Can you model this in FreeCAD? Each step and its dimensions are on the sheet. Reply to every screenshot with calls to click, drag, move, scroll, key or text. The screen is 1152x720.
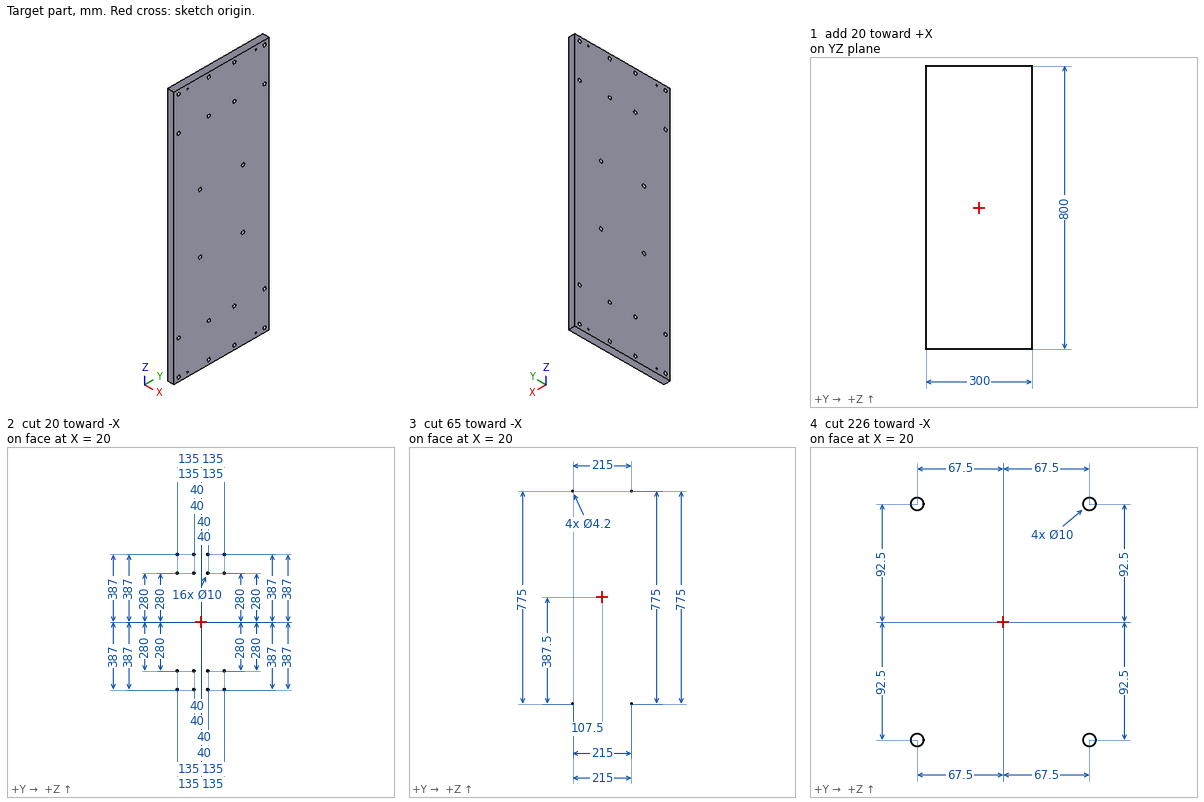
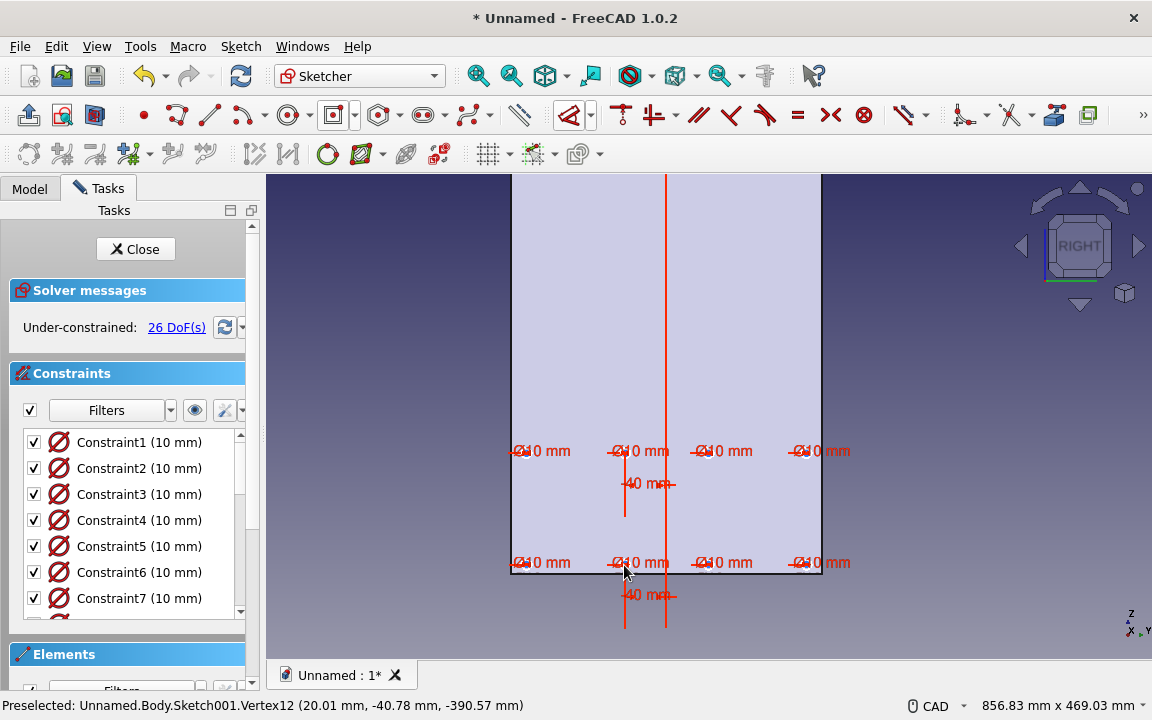
click(709, 565)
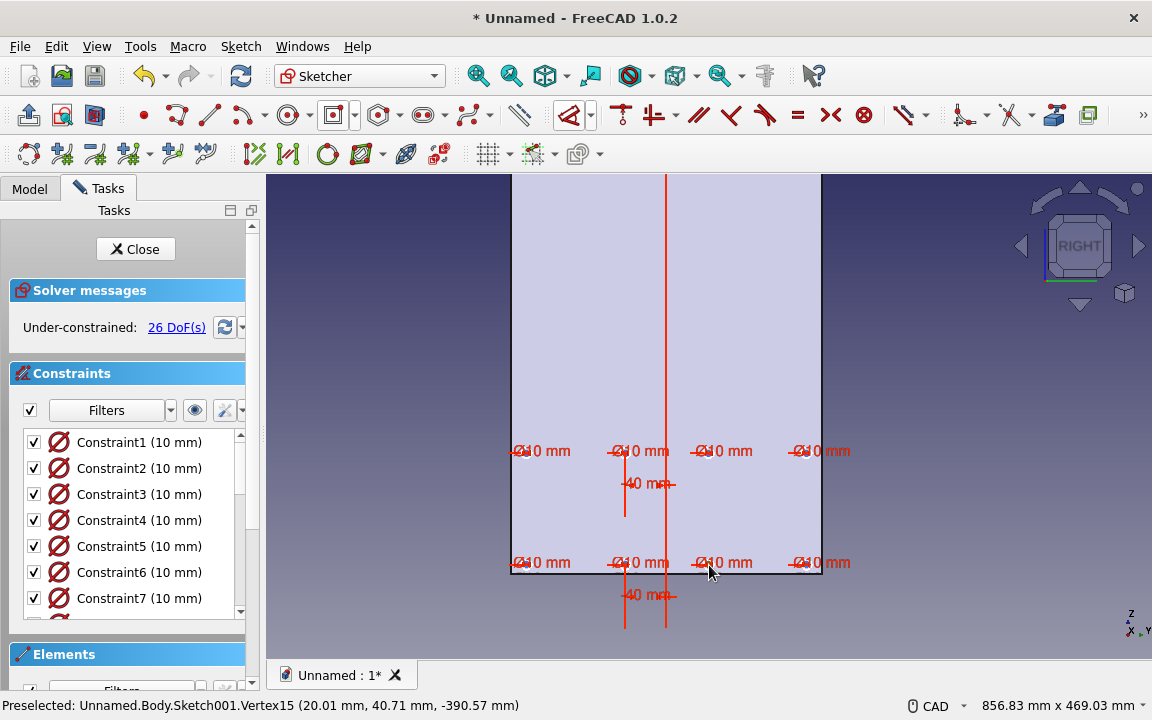
key(l)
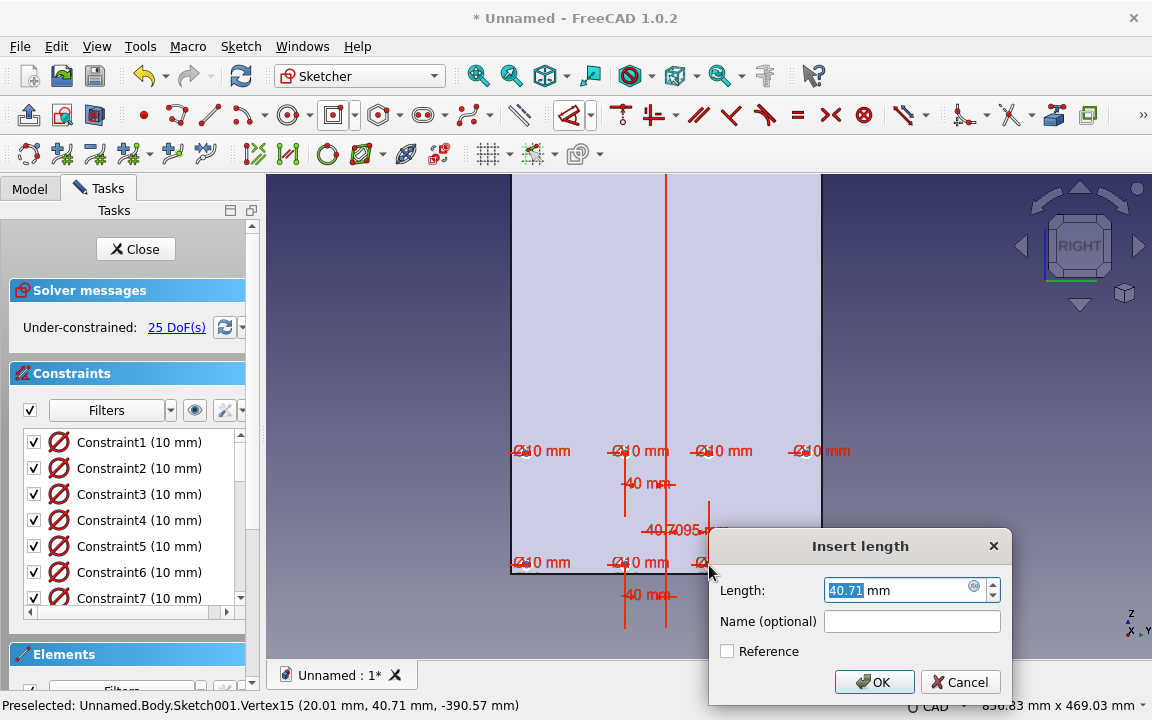
text(40)
key(Return)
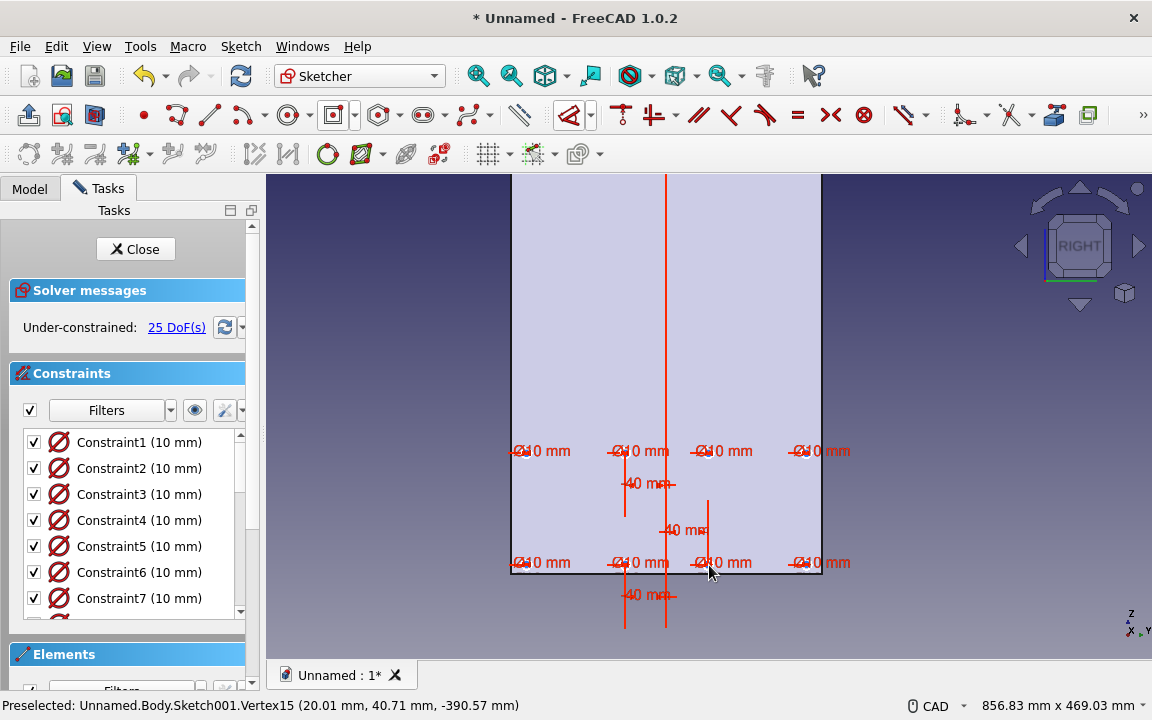
click(709, 453)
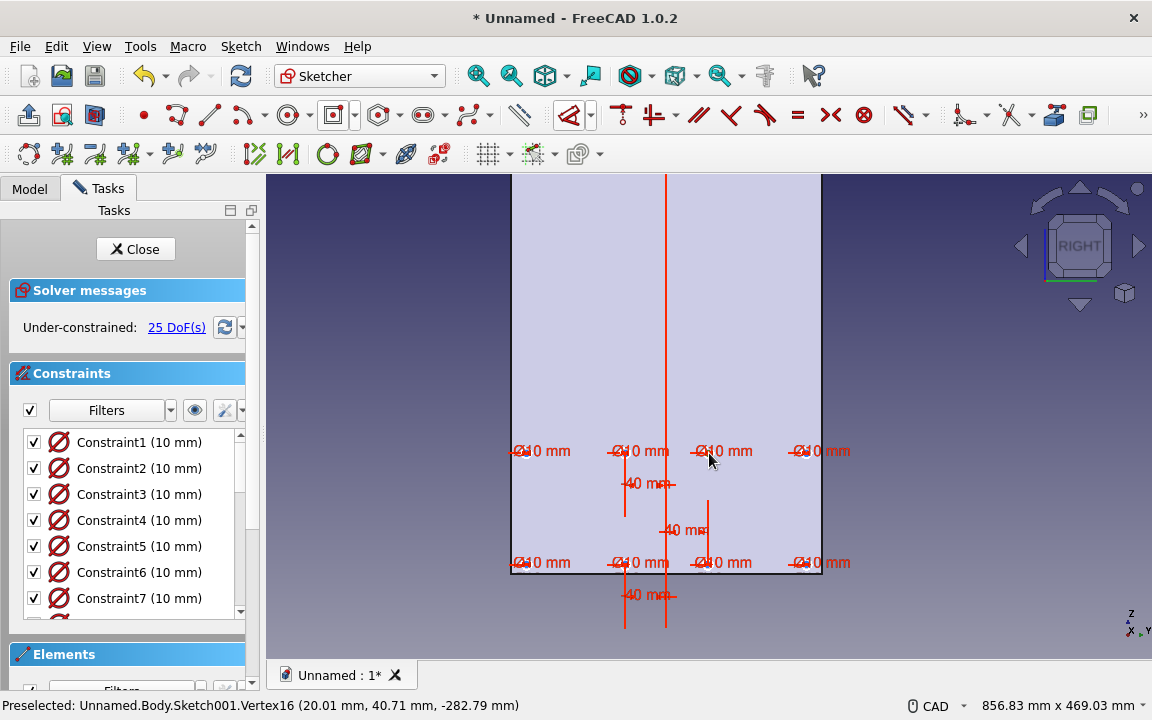
key(l)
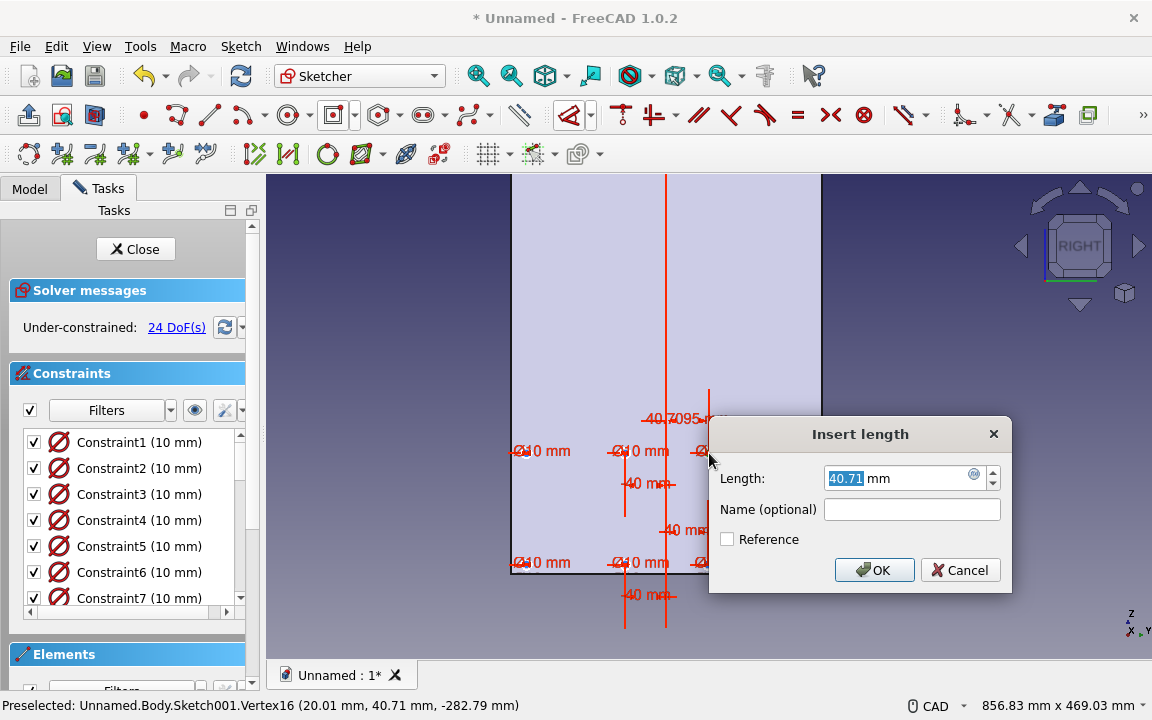
text(40)
key(Return)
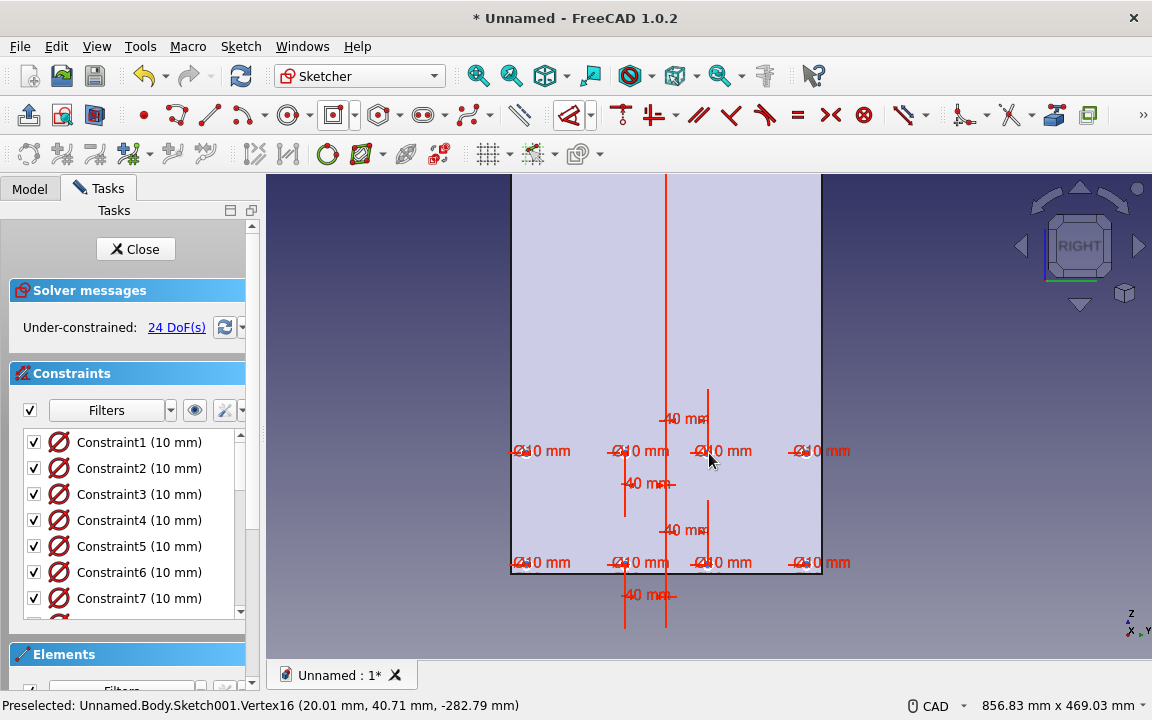
scroll(625, 565, down, 5)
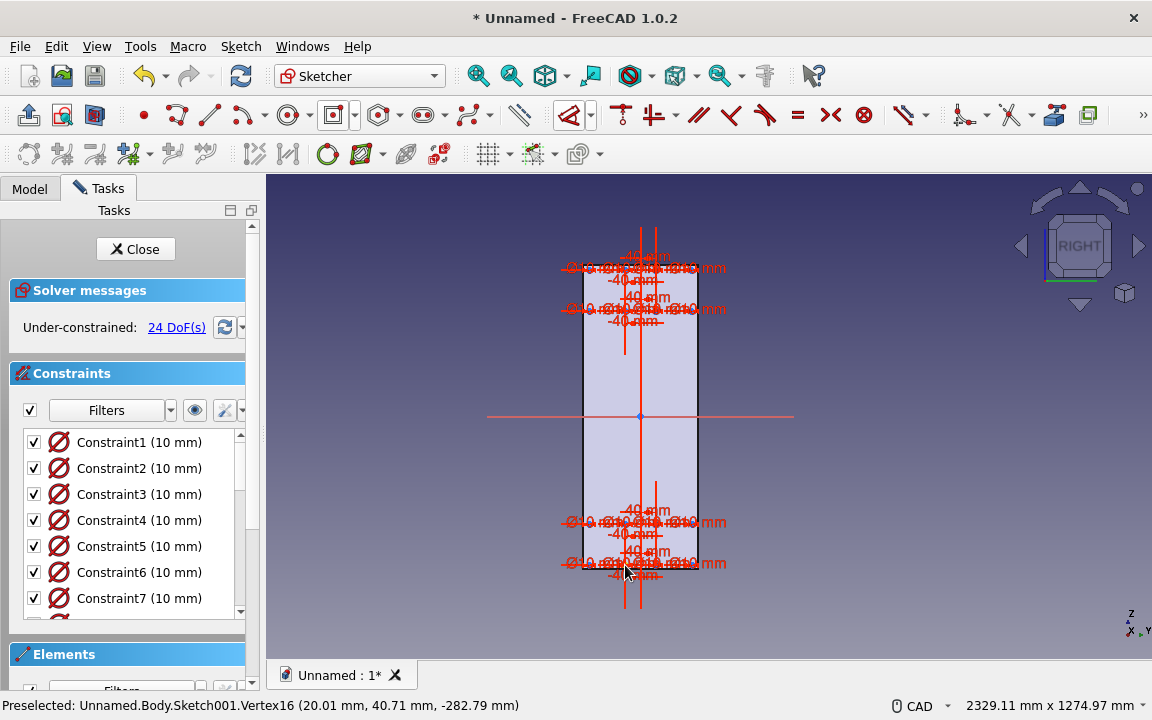
click(692, 270)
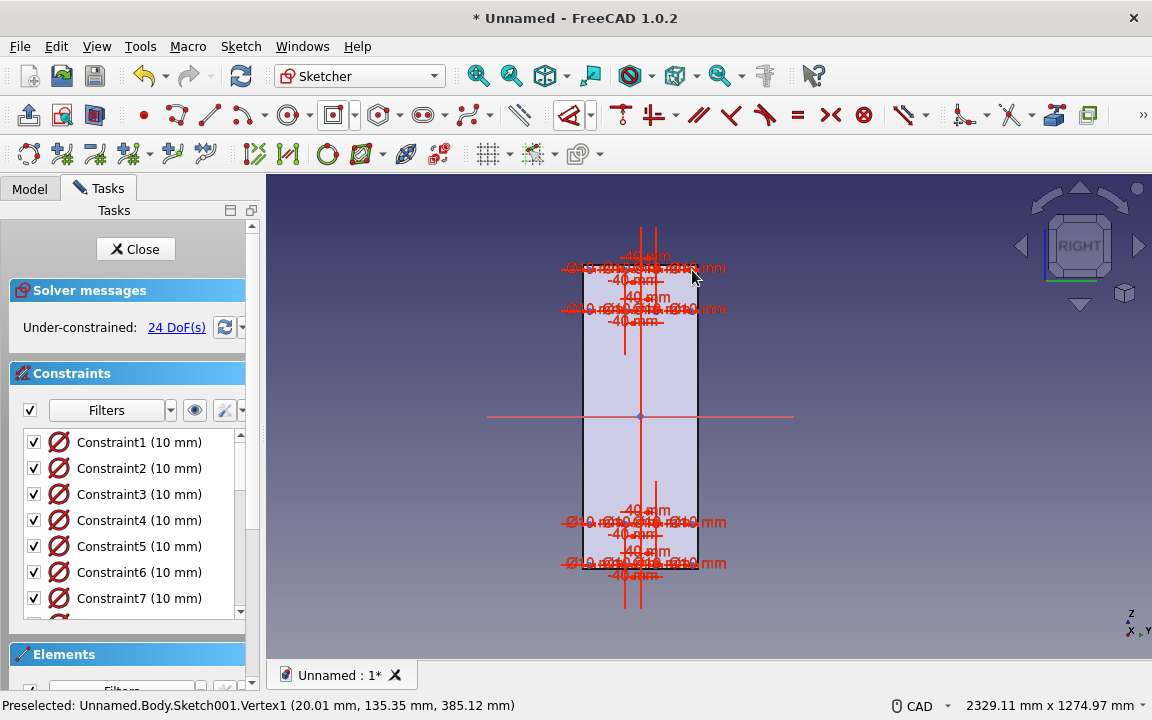
key(l)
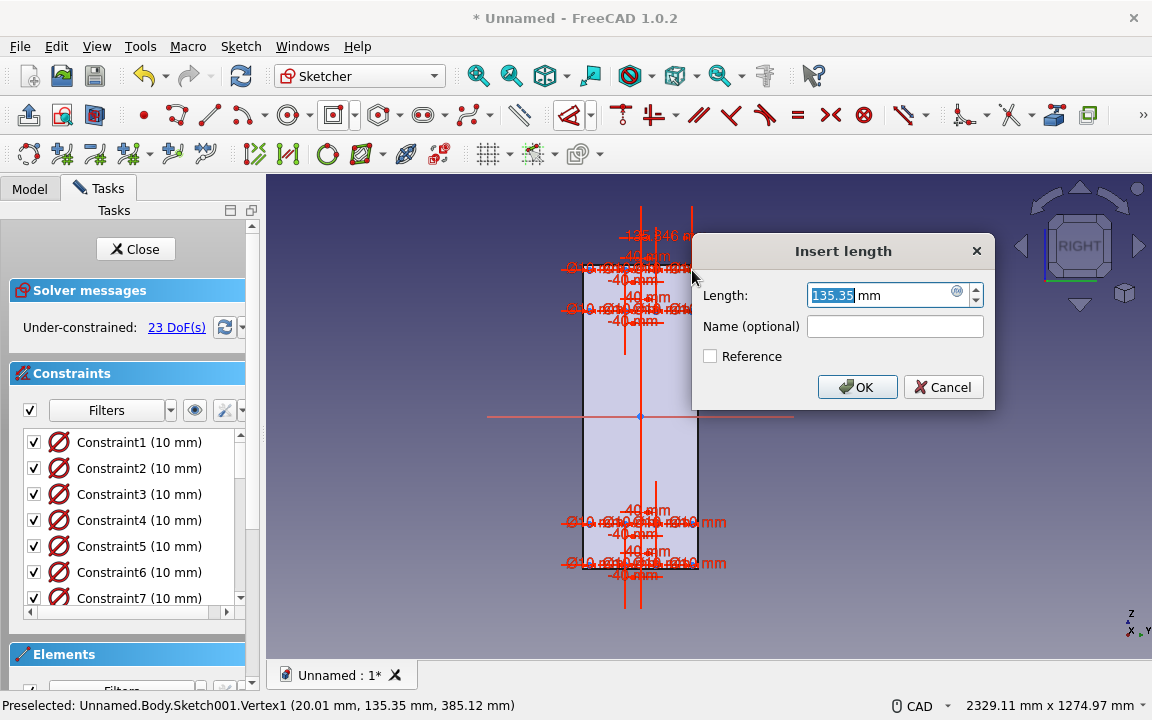
text(135)
key(Return)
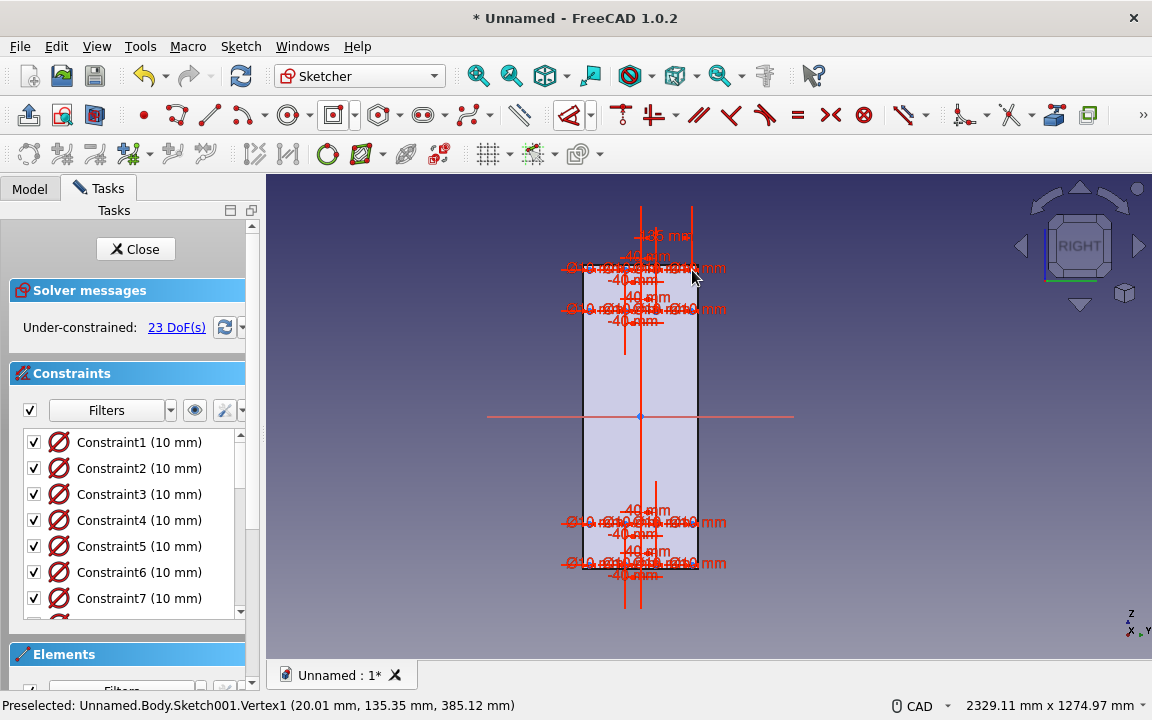
click(692, 270)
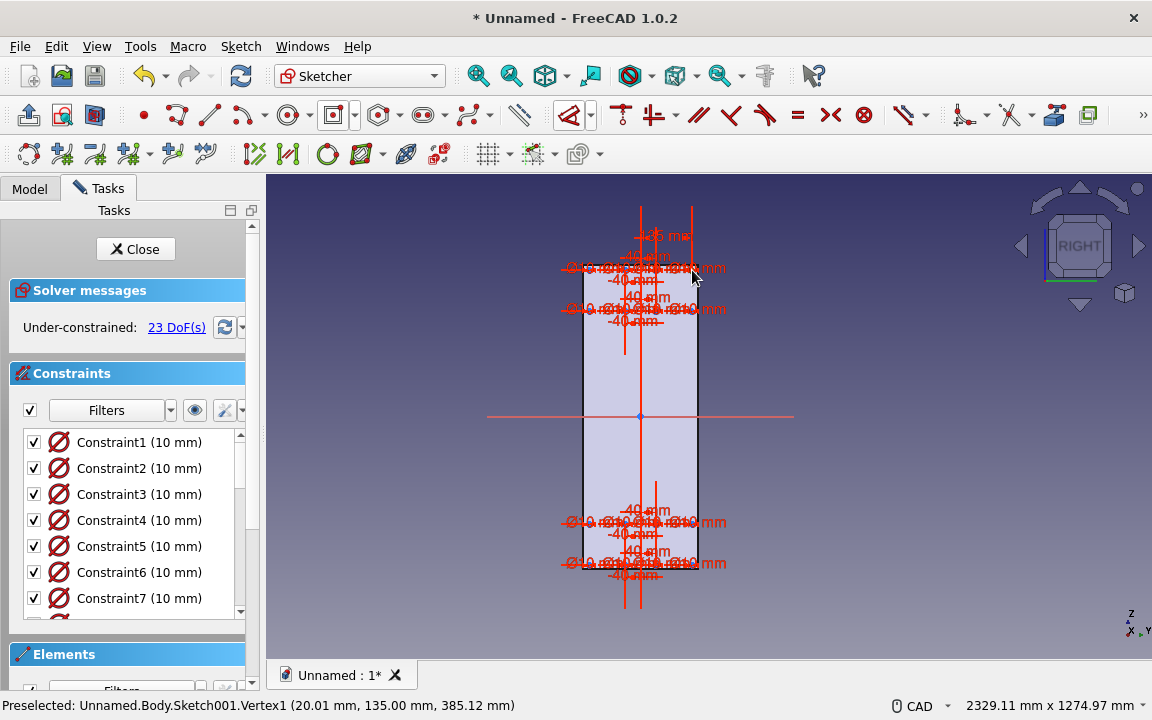
click(590, 116)